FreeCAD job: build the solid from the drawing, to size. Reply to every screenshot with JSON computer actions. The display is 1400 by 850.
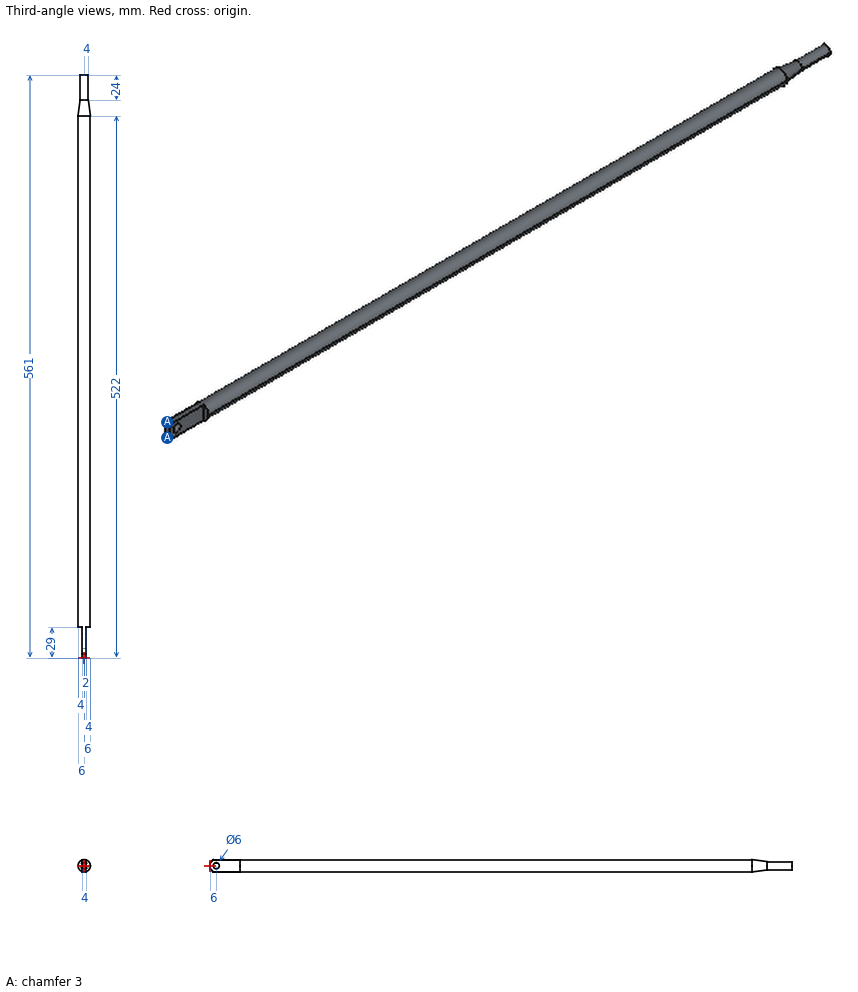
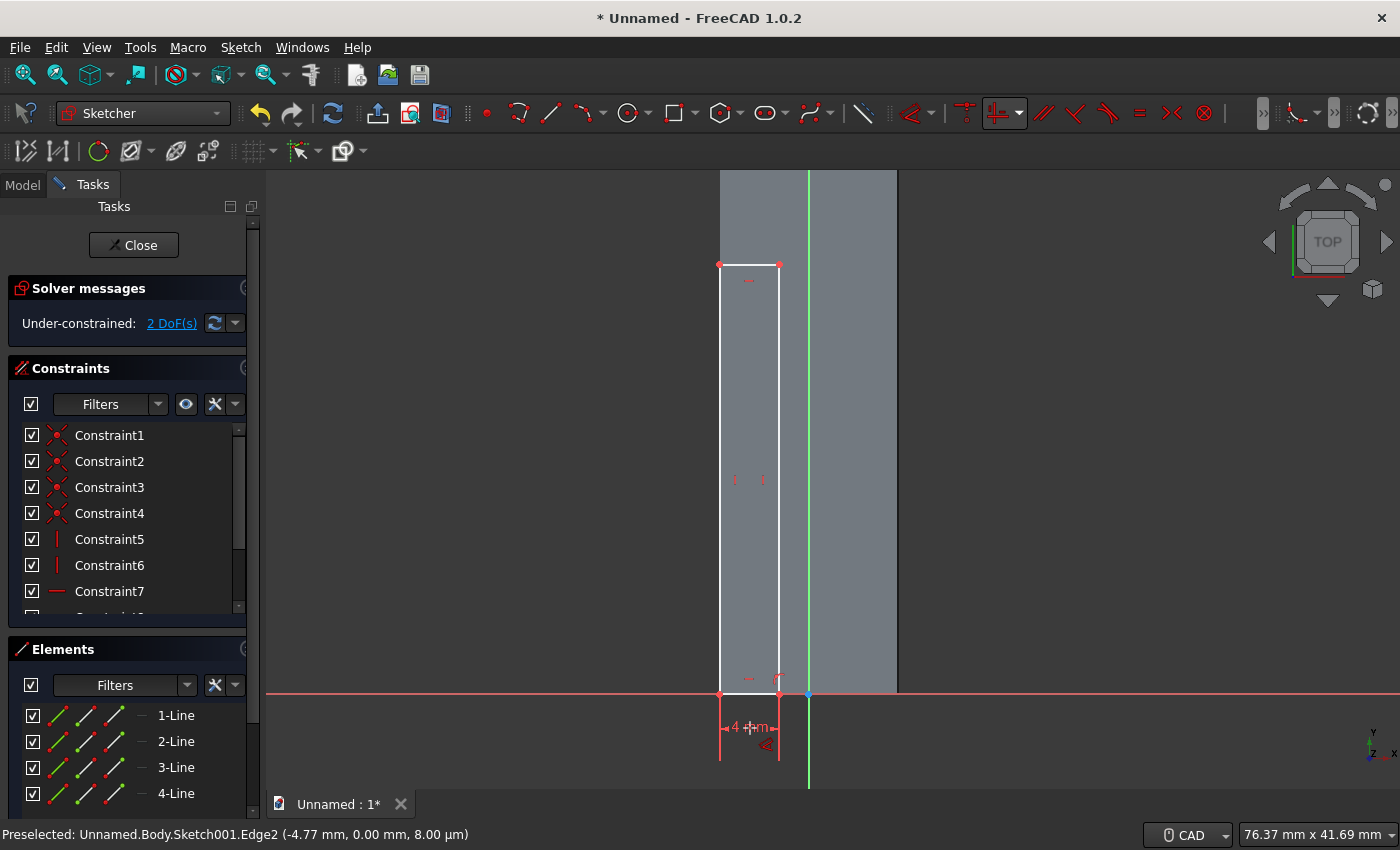
{"action": "left_click", "coordinate": [720, 394]}
{"action": "left_click", "coordinate": [686, 480]}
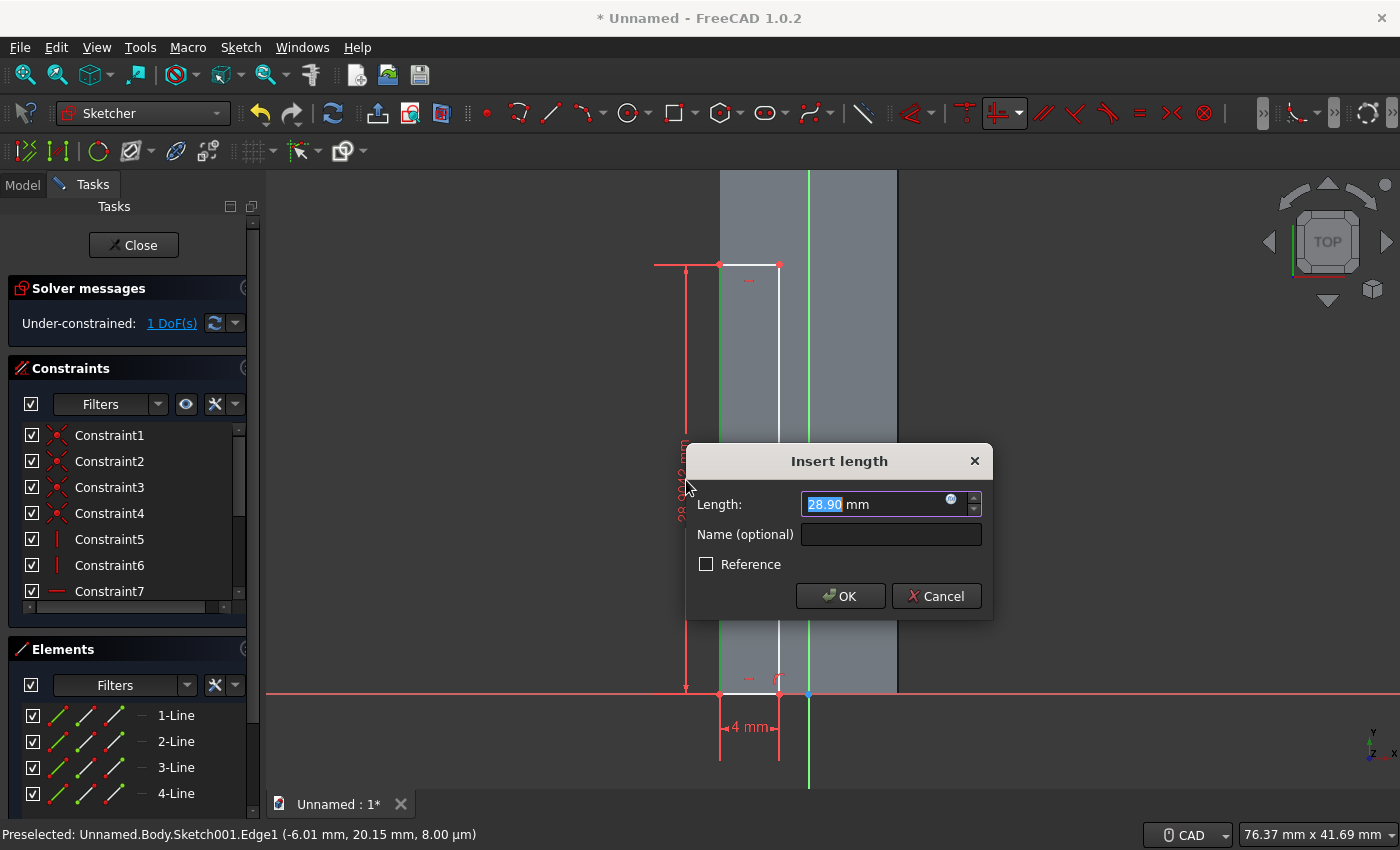
{"action": "type", "text": "29"}
{"action": "key", "text": "Return"}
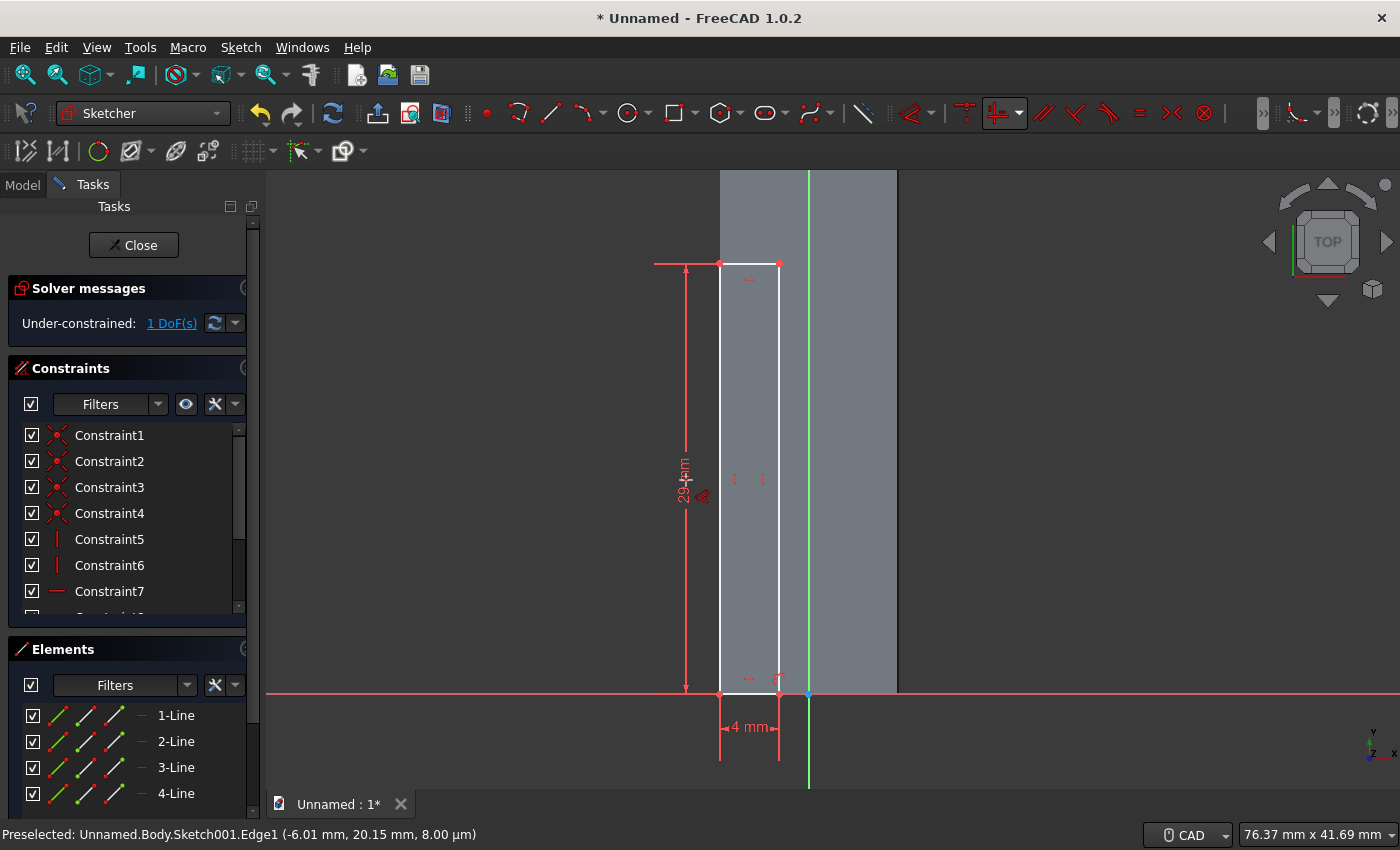
{"action": "left_click", "coordinate": [720, 264]}
{"action": "left_click", "coordinate": [764, 230]}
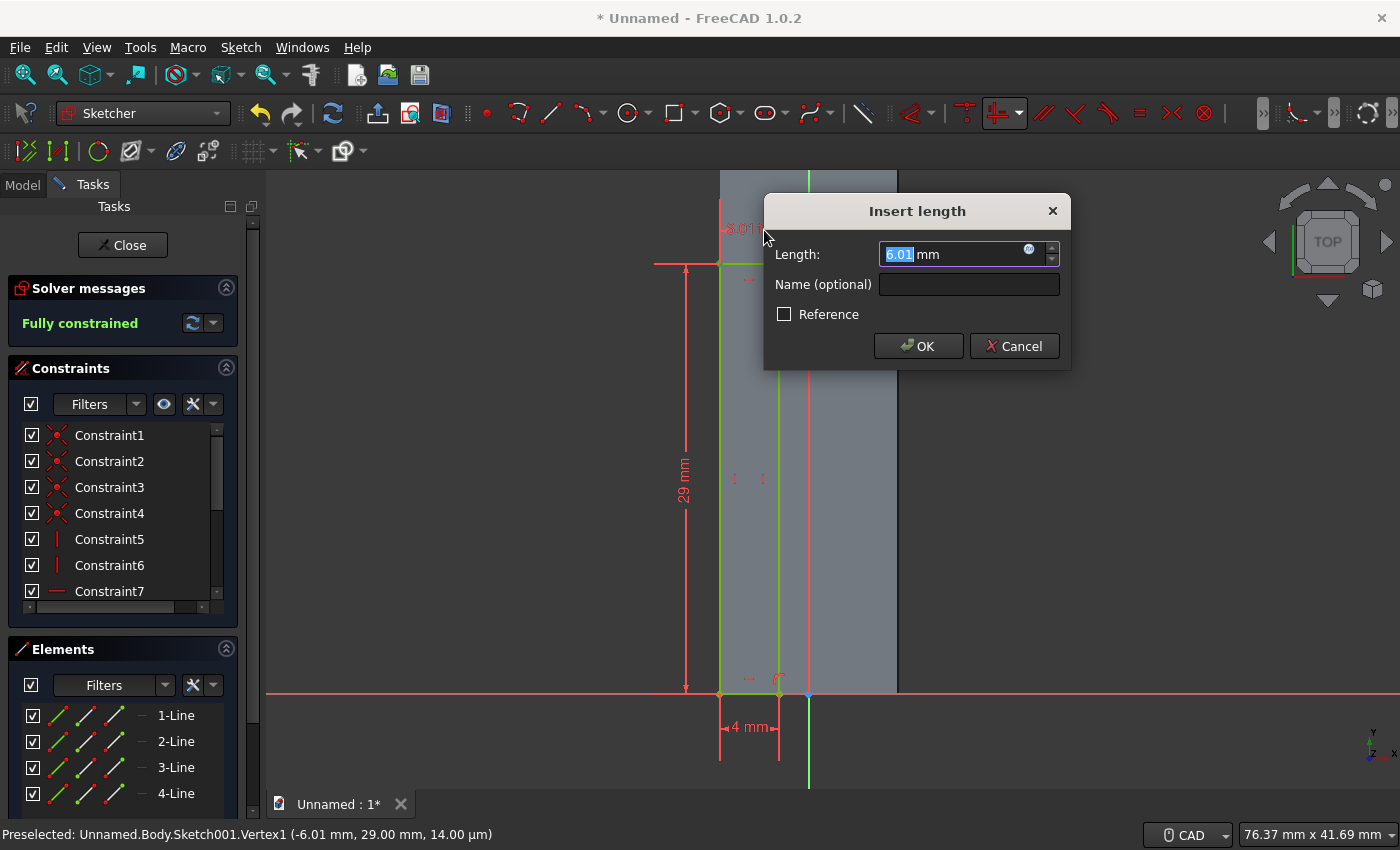
{"action": "type", "text": "6"}
{"action": "key", "text": "Return"}
{"action": "key", "text": "Escape"}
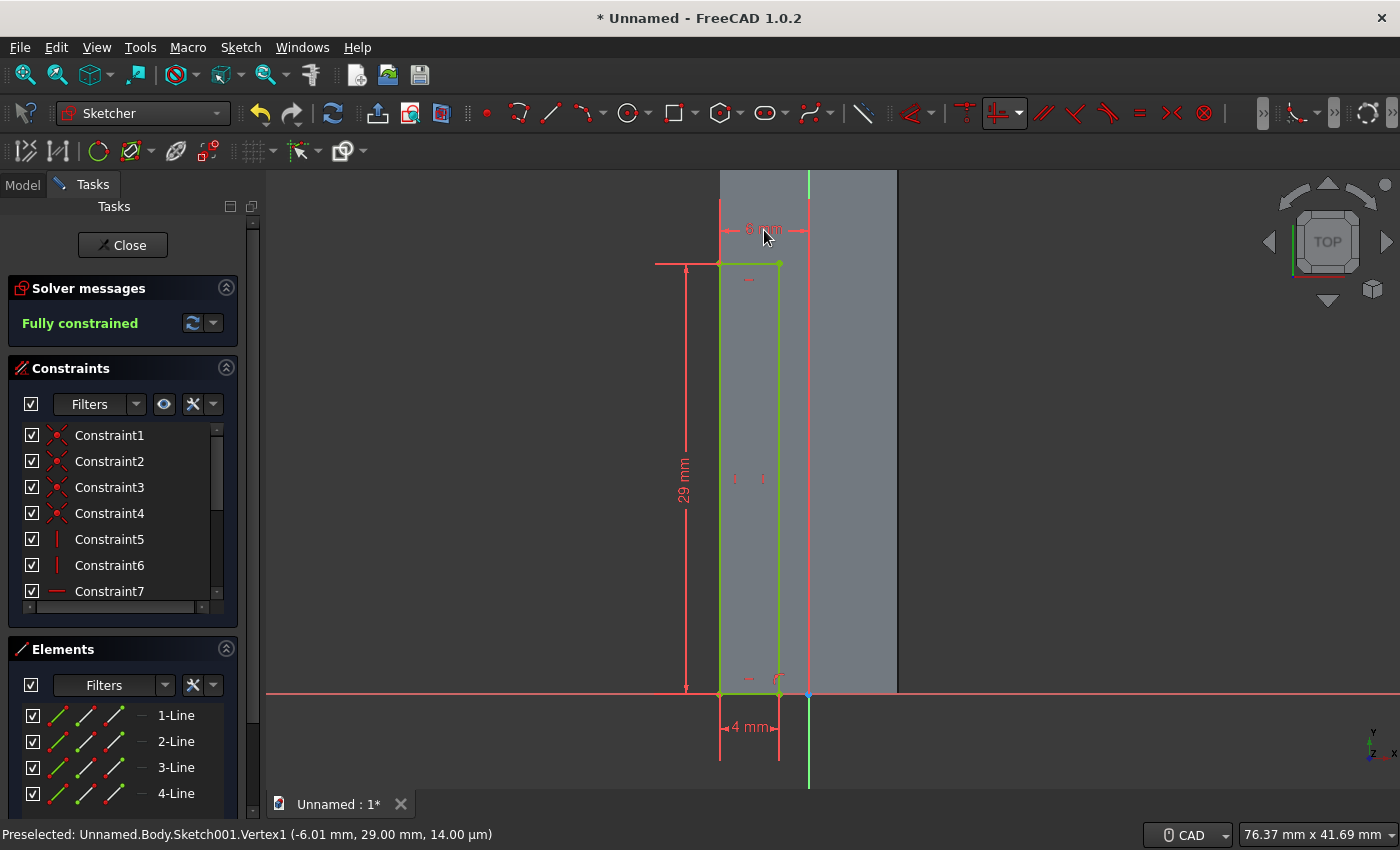
{"action": "left_click", "coordinate": [123, 245]}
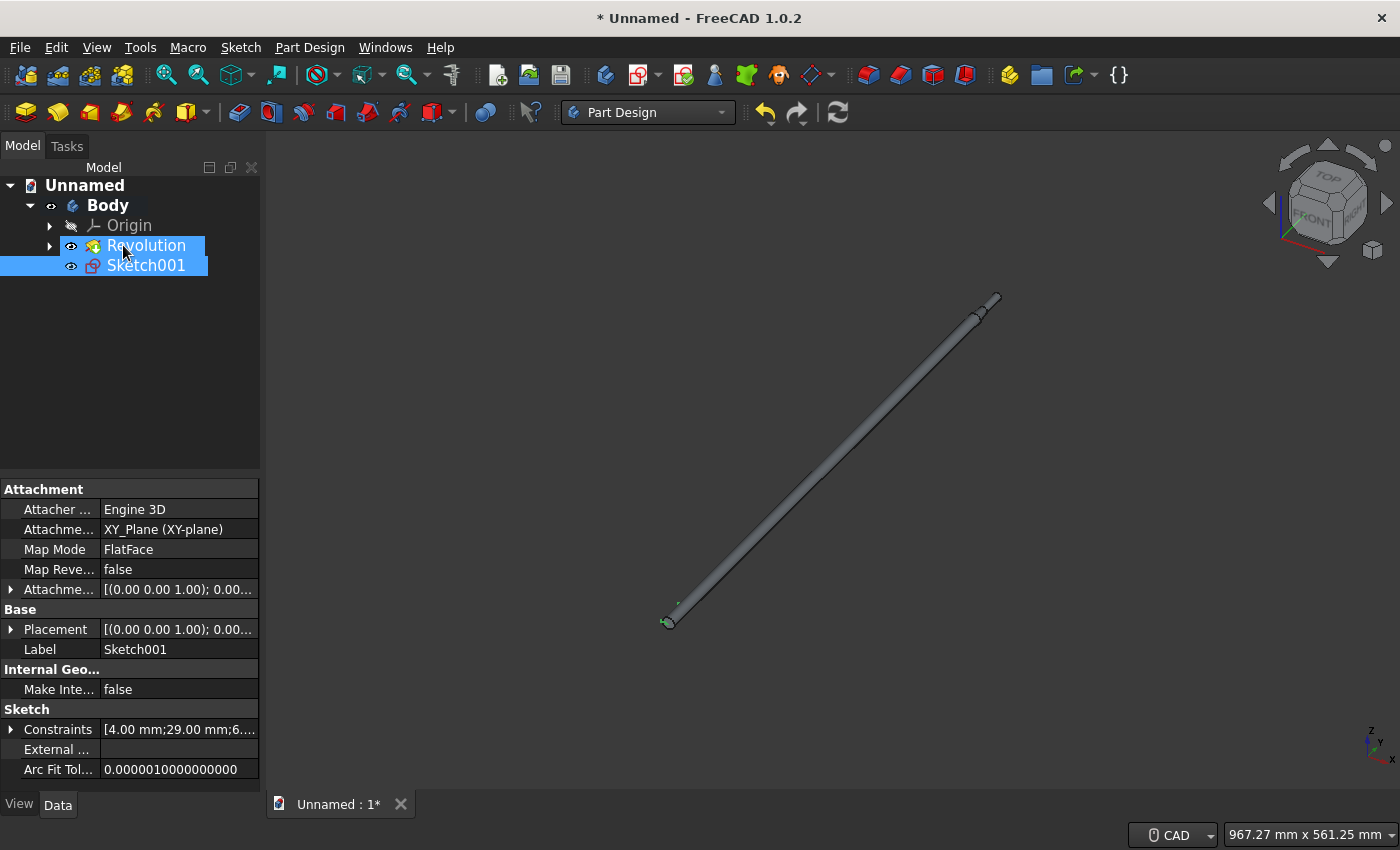
{"action": "left_click", "coordinate": [240, 112]}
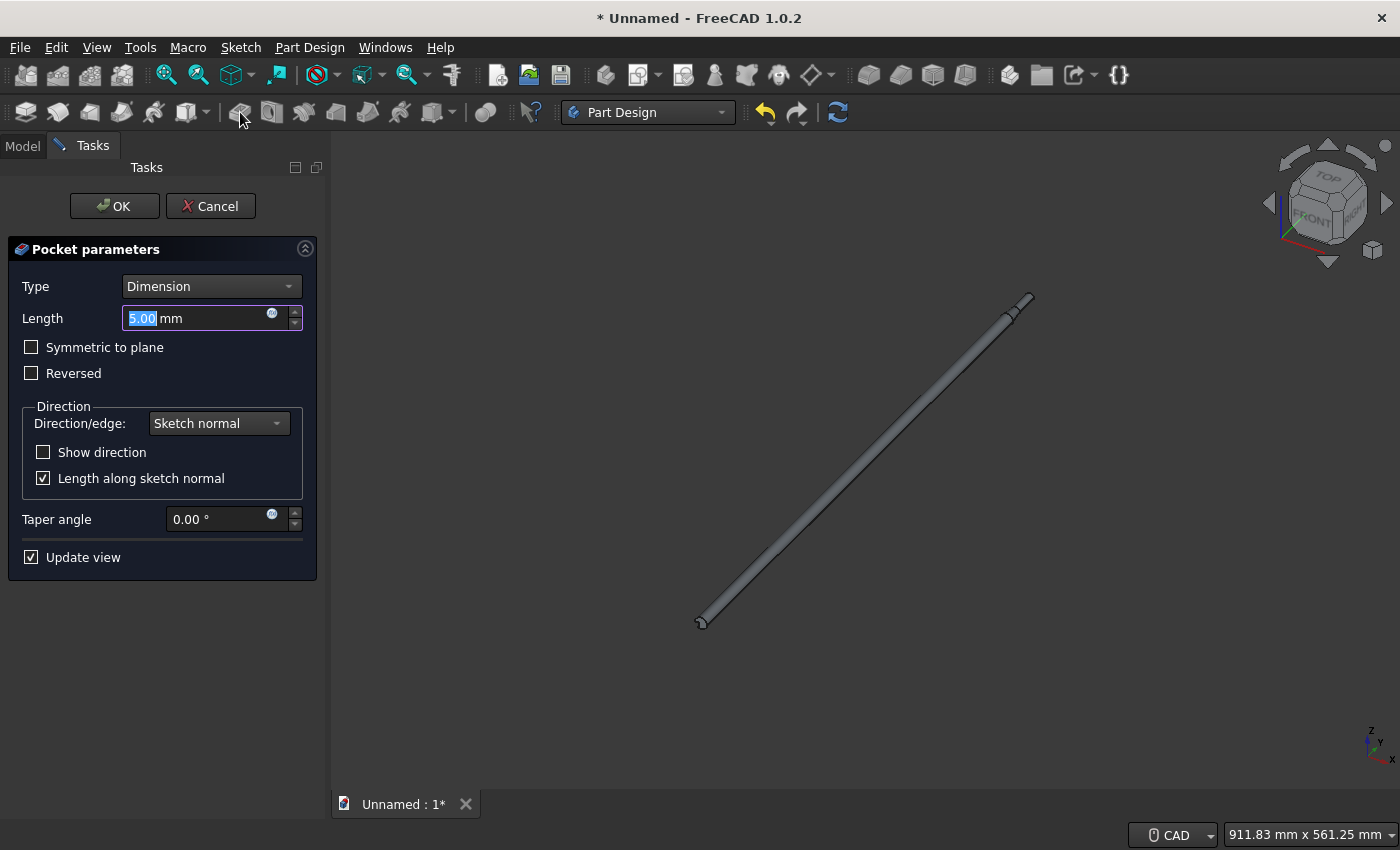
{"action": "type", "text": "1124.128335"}
{"action": "key", "text": "Tab"}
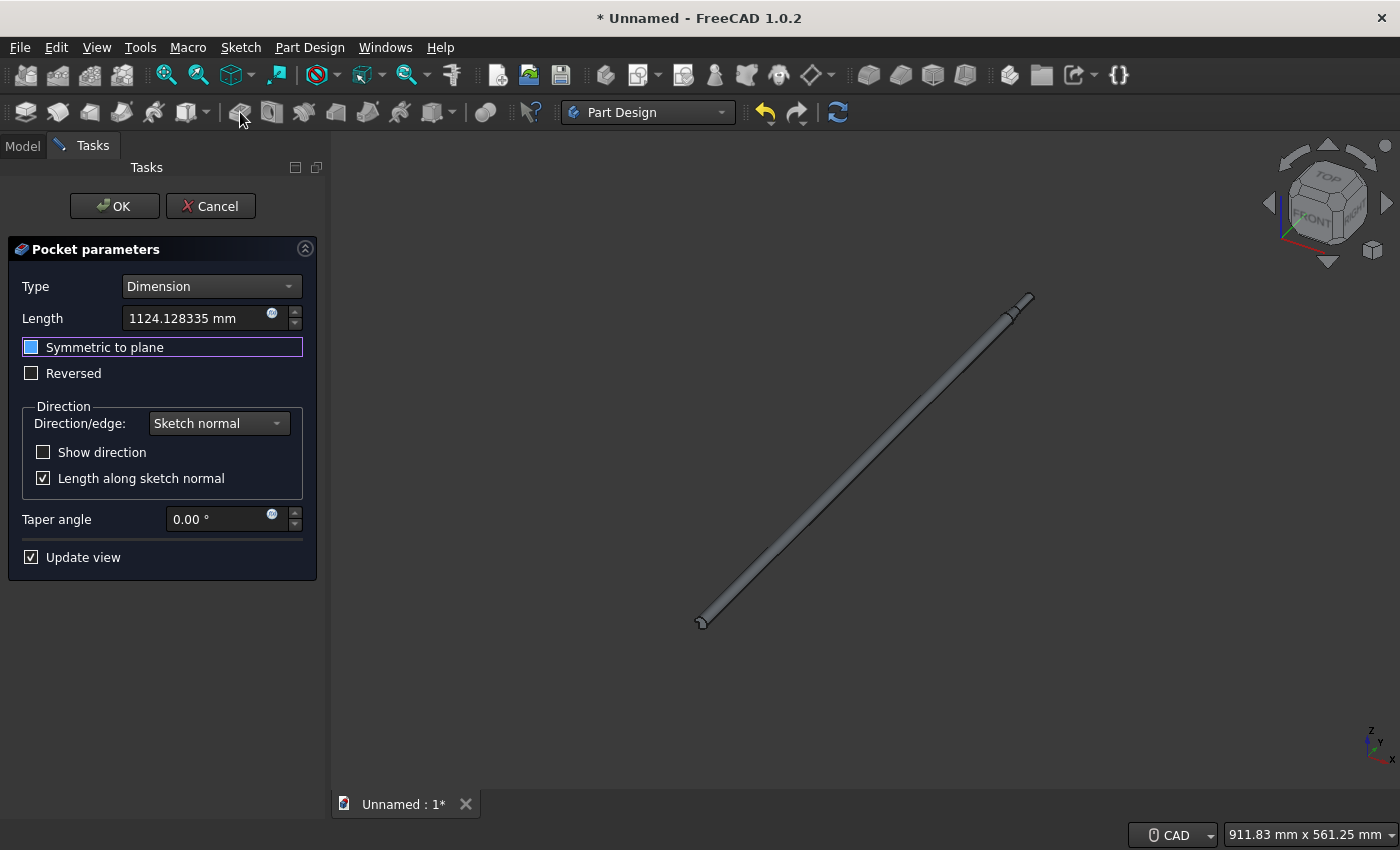
{"action": "left_click", "coordinate": [30, 347]}